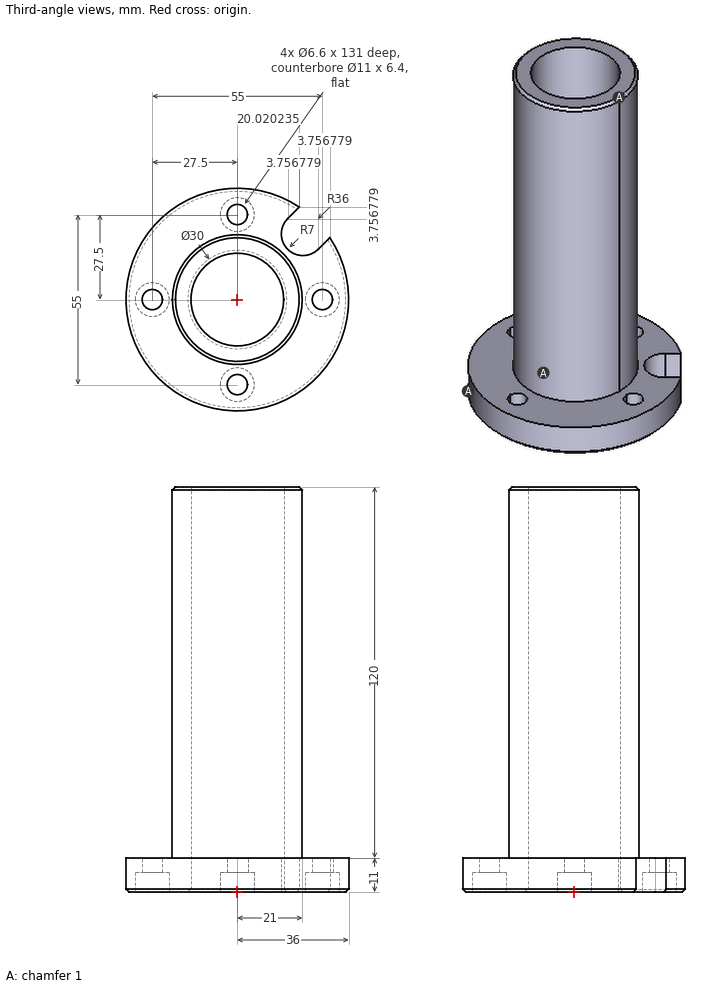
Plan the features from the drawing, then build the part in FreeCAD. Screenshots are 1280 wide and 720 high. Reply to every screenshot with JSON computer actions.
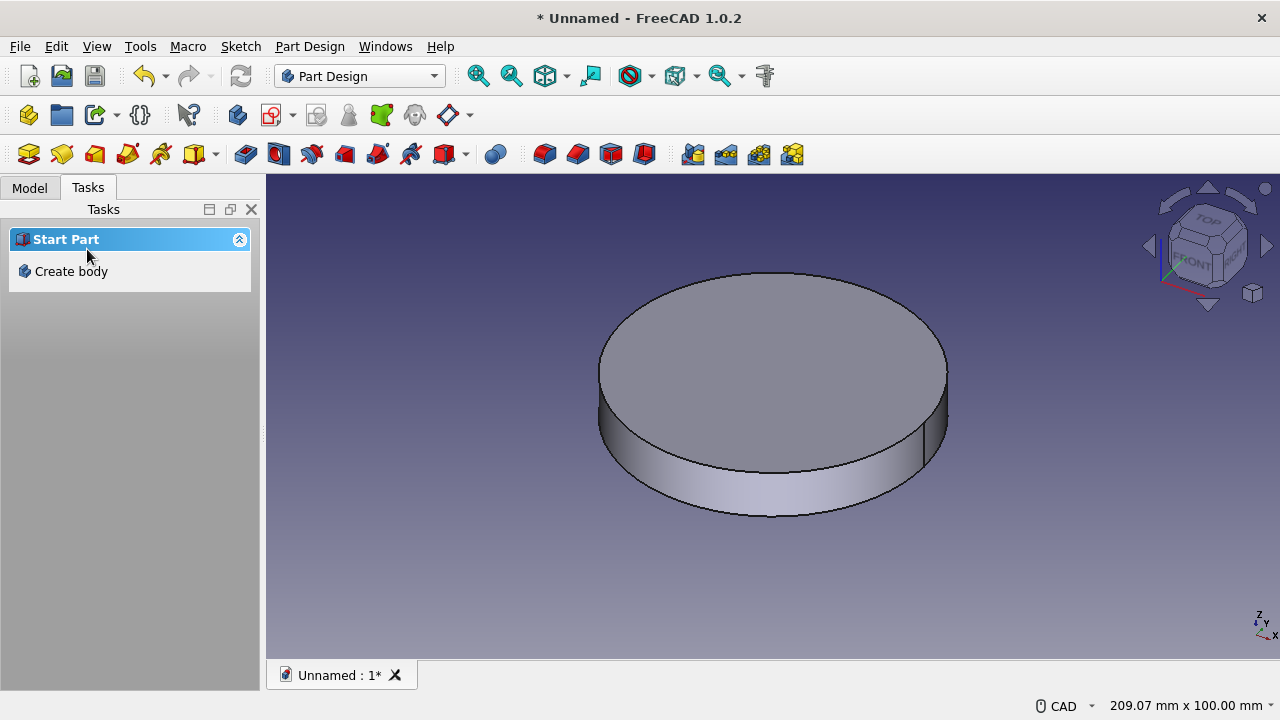
{"action": "left_click", "coordinate": [773, 372]}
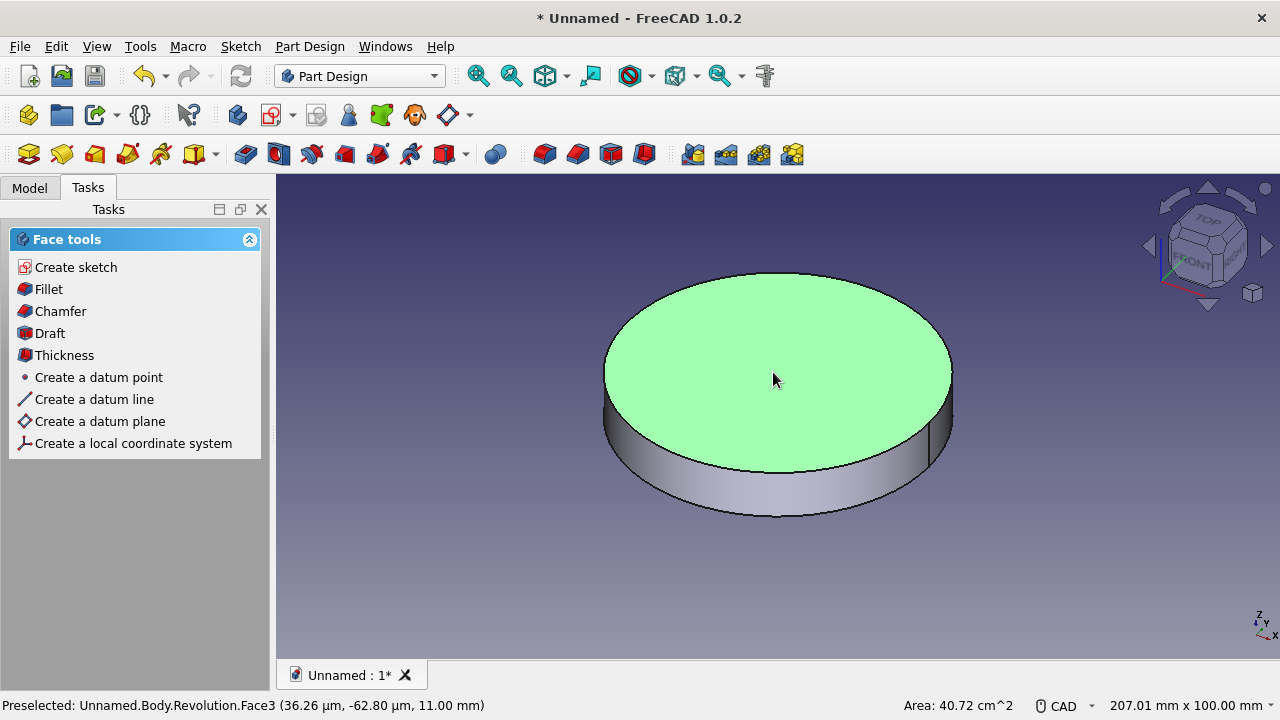
{"action": "left_click", "coordinate": [270, 116]}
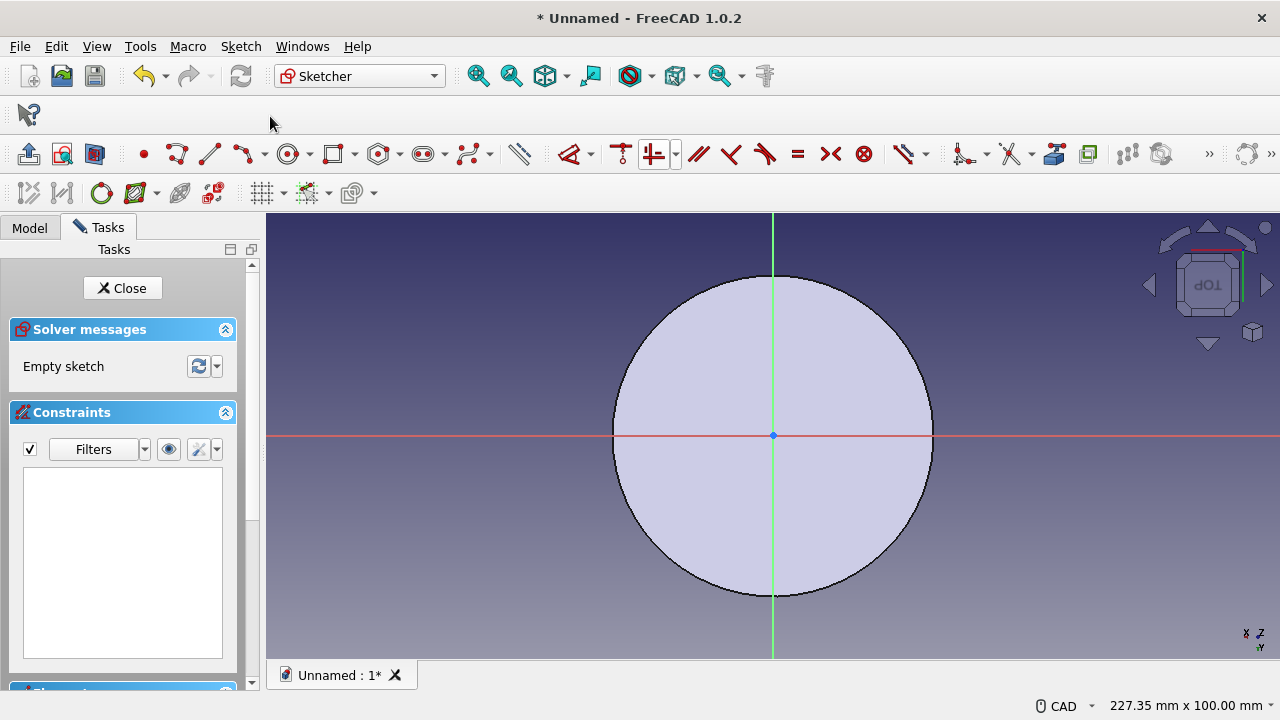
{"action": "scroll", "coordinate": [708, 557], "scroll_direction": "up", "scroll_amount": 4}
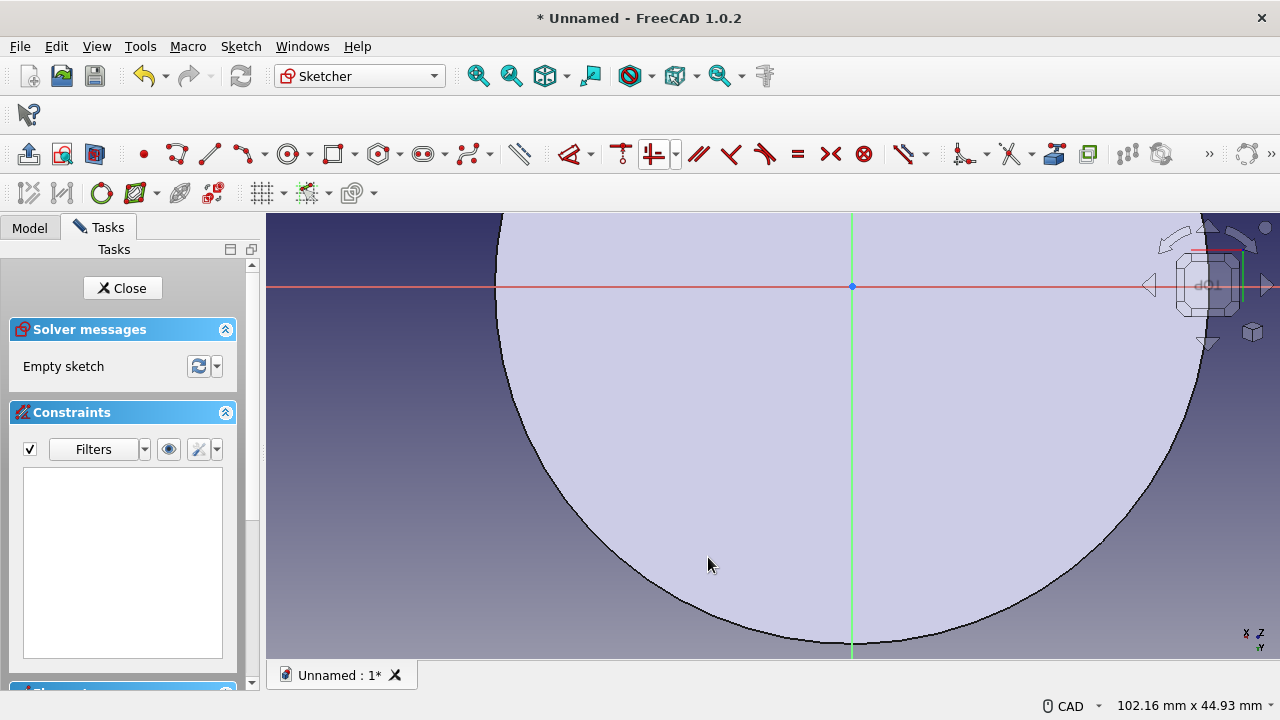
{"action": "left_click", "coordinate": [210, 154]}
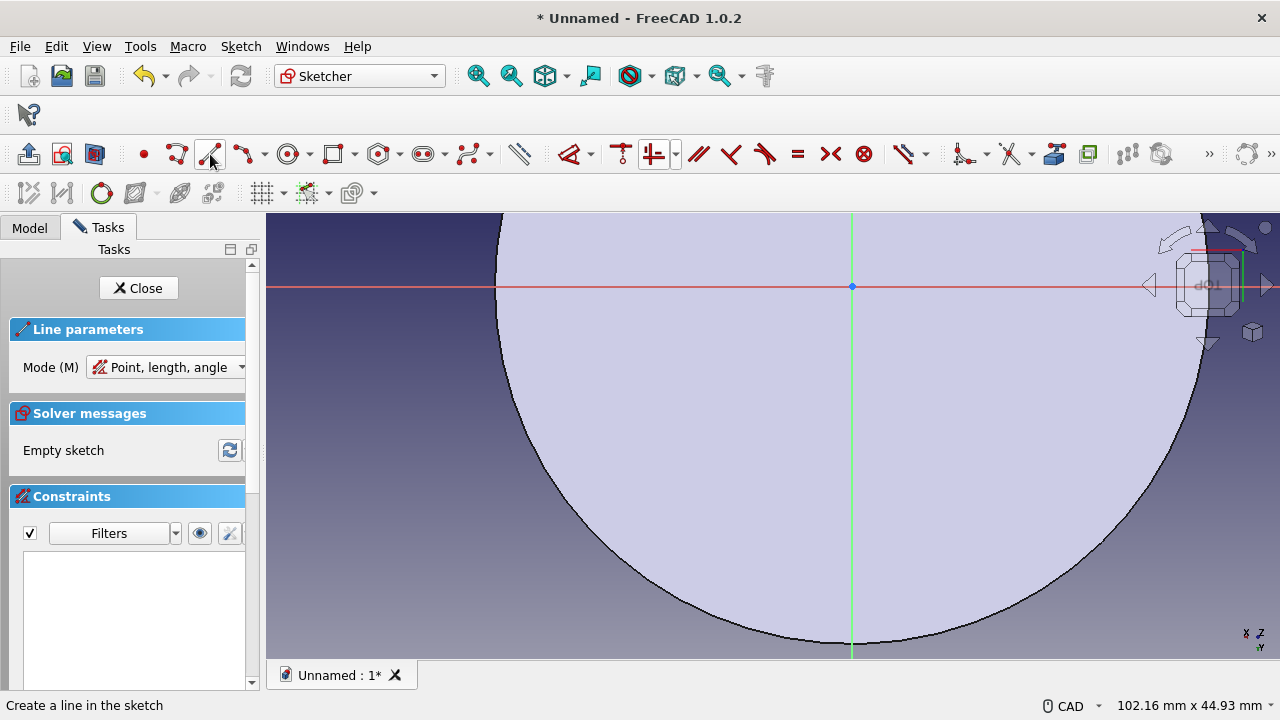
{"action": "left_click", "coordinate": [653, 584]}
{"action": "left_click", "coordinate": [691, 546]}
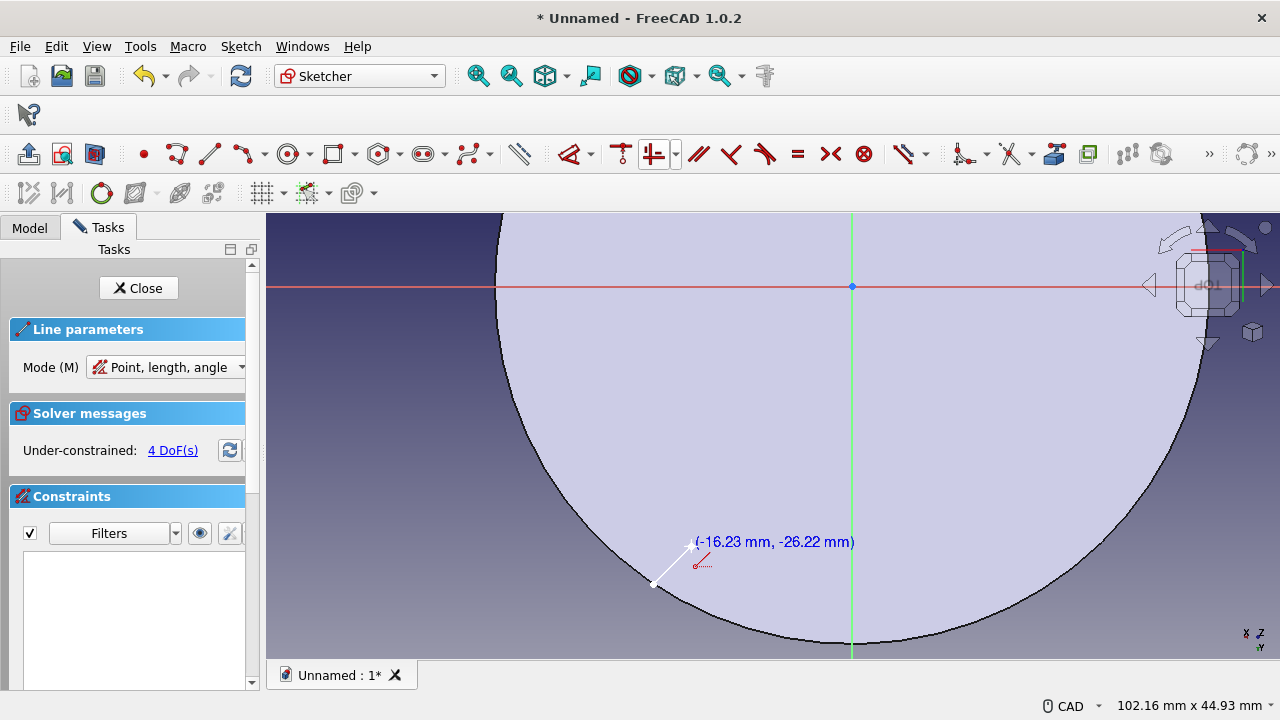
{"action": "left_click", "coordinate": [592, 448]}
{"action": "left_click", "coordinate": [555, 485]}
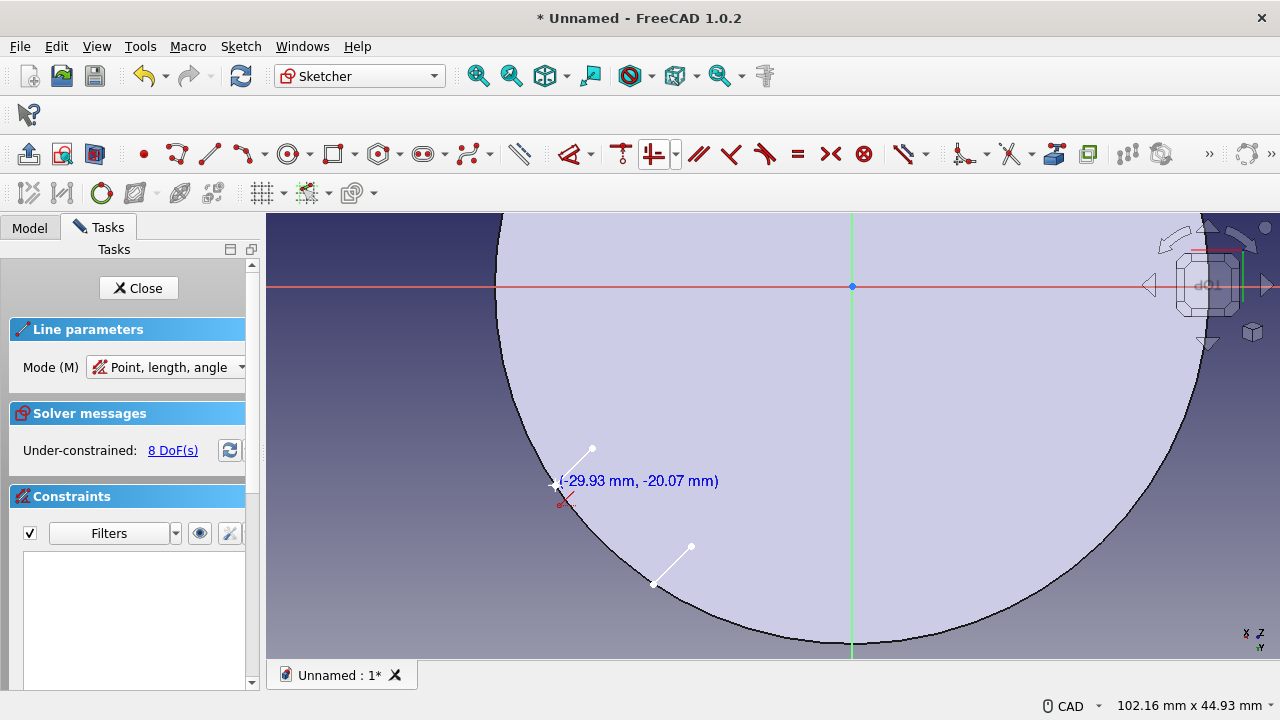
{"action": "key", "text": "g 3 a"}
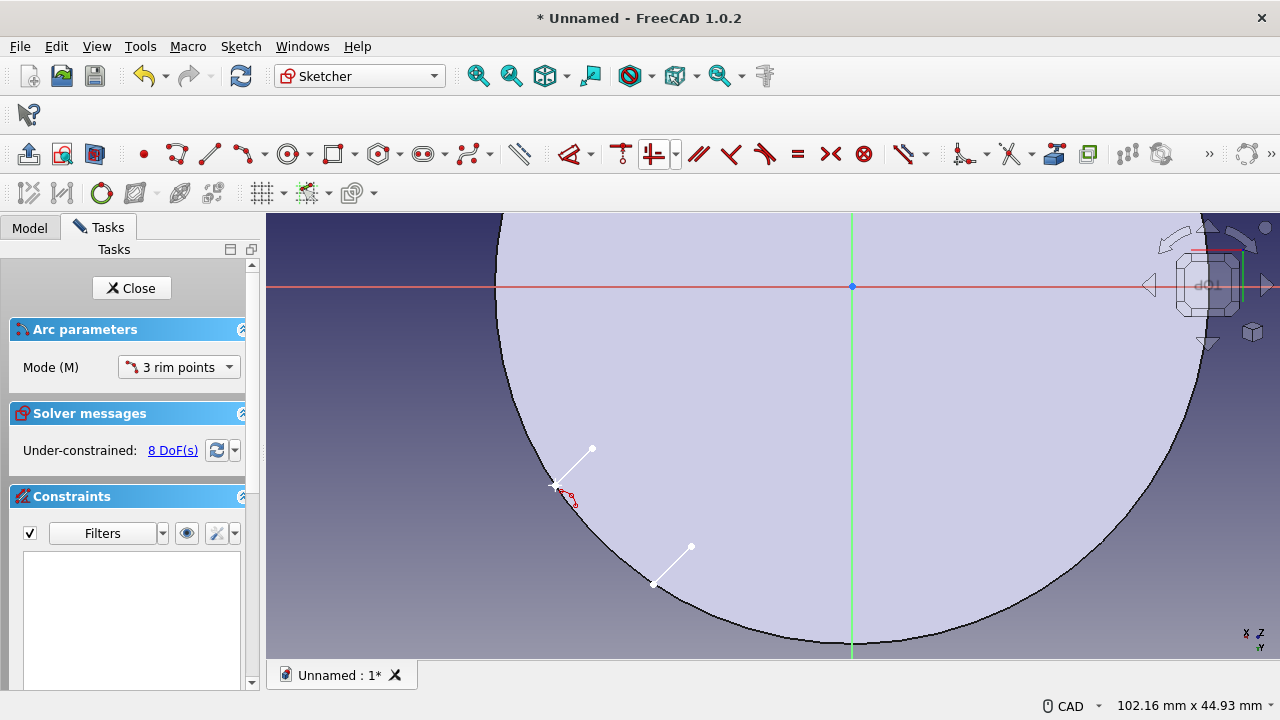
{"action": "left_click", "coordinate": [691, 547]}
{"action": "left_click", "coordinate": [592, 449]}
{"action": "left_click", "coordinate": [691, 448]}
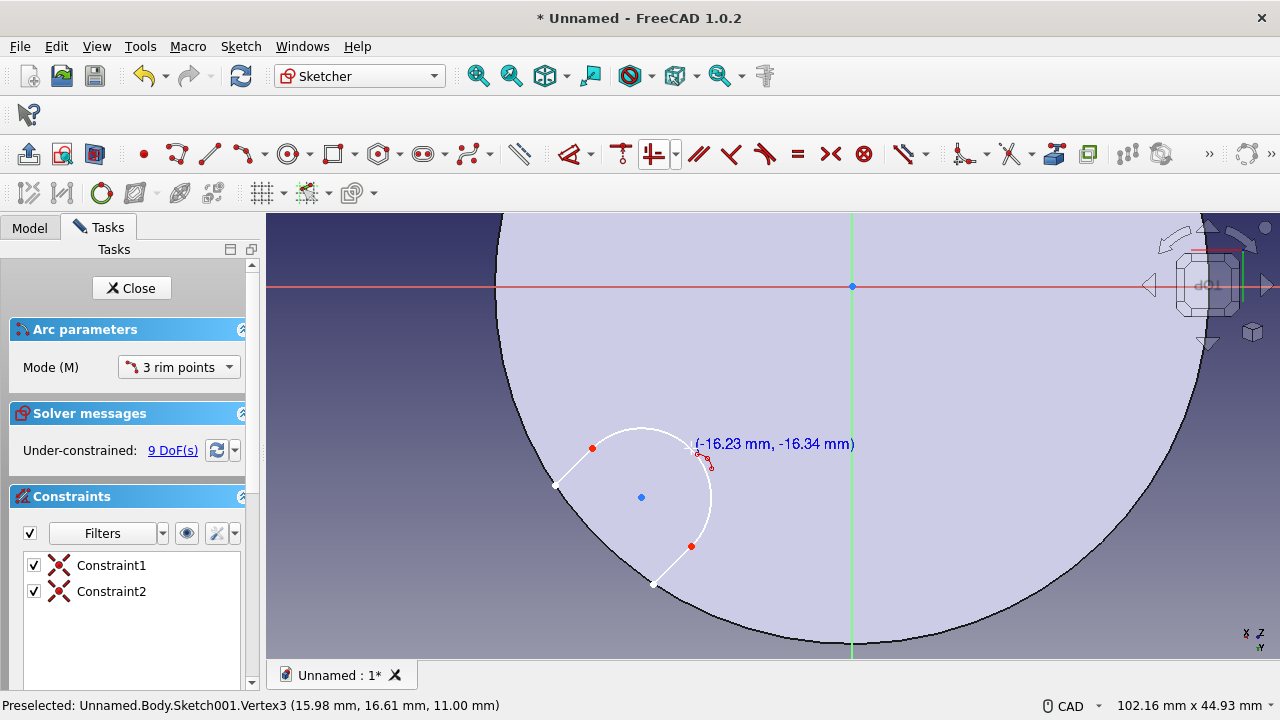
{"action": "left_click", "coordinate": [555, 486]}
{"action": "left_click", "coordinate": [653, 585]}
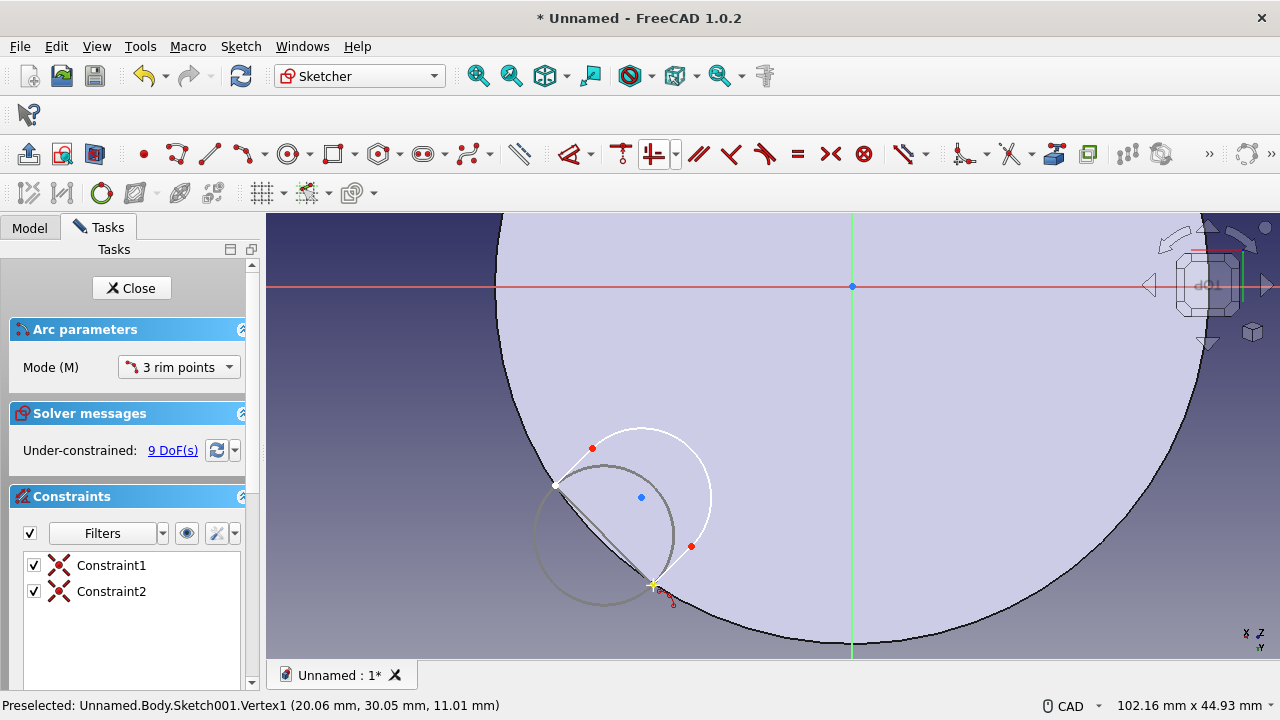
{"action": "scroll", "coordinate": [599, 539], "scroll_direction": "up", "scroll_amount": 5}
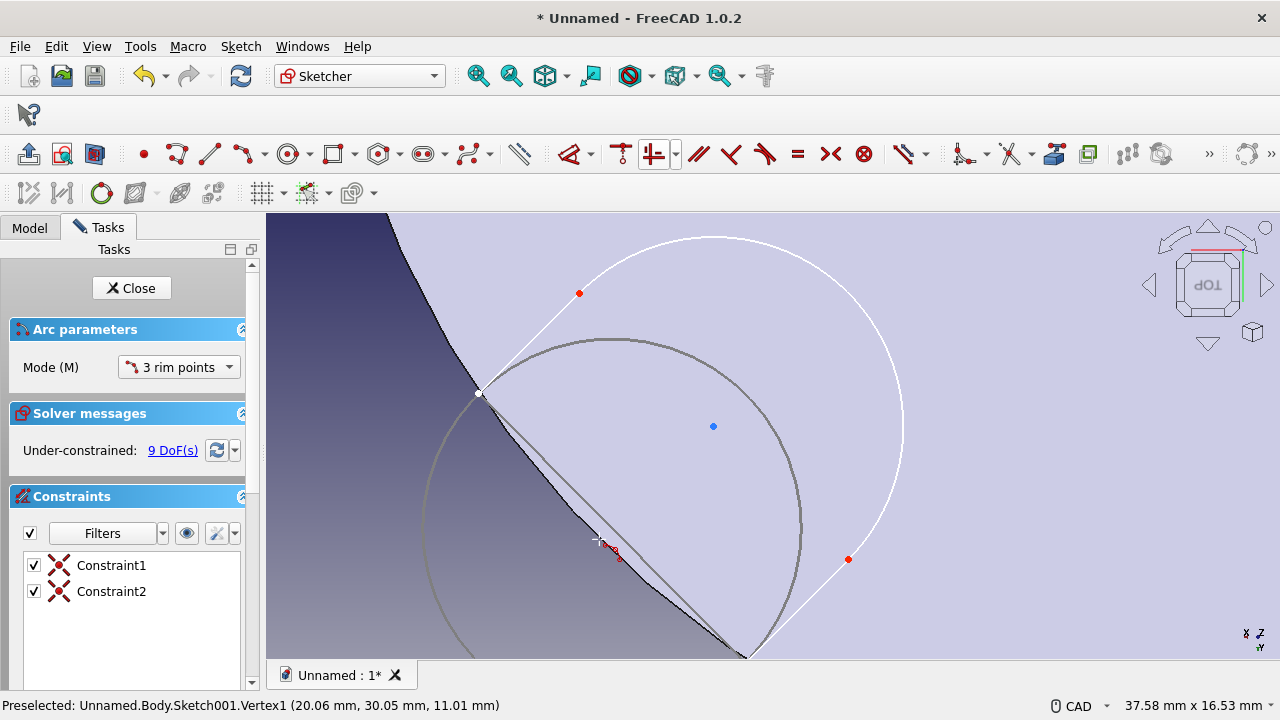
{"action": "left_click", "coordinate": [600, 539]}
{"action": "key", "text": "Escape"}